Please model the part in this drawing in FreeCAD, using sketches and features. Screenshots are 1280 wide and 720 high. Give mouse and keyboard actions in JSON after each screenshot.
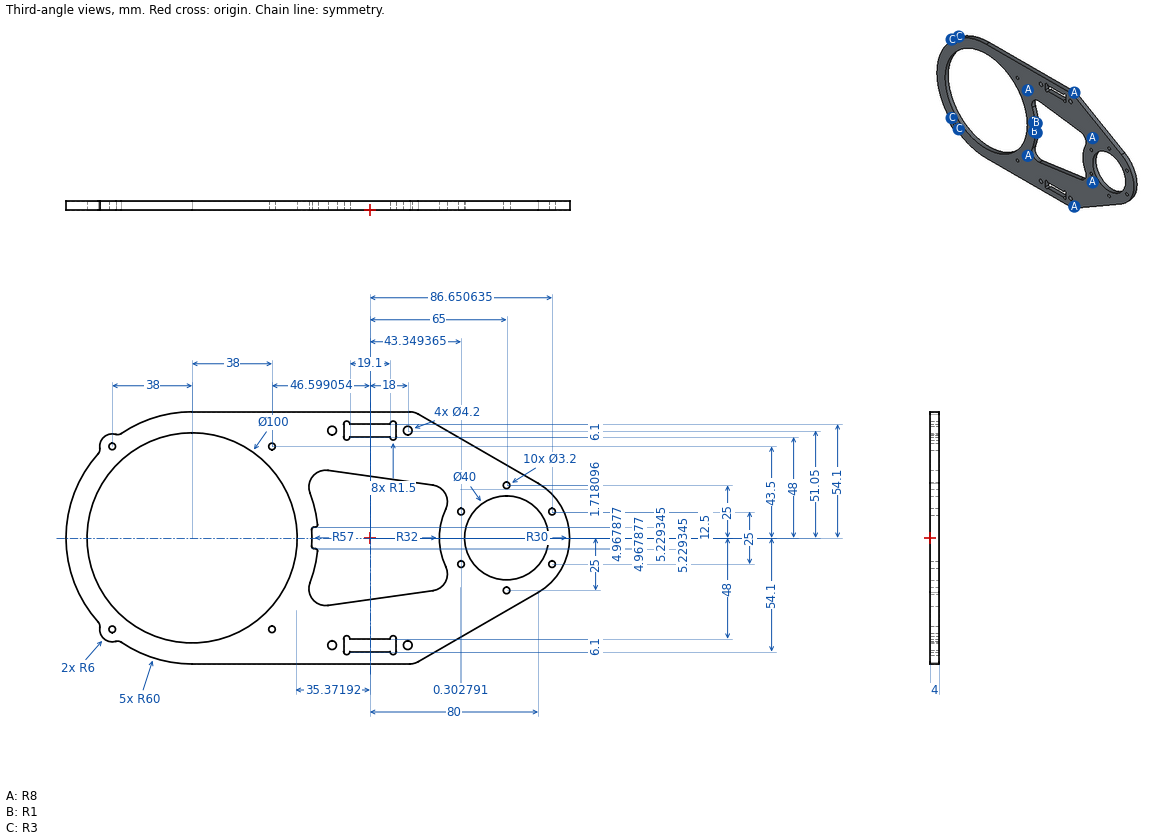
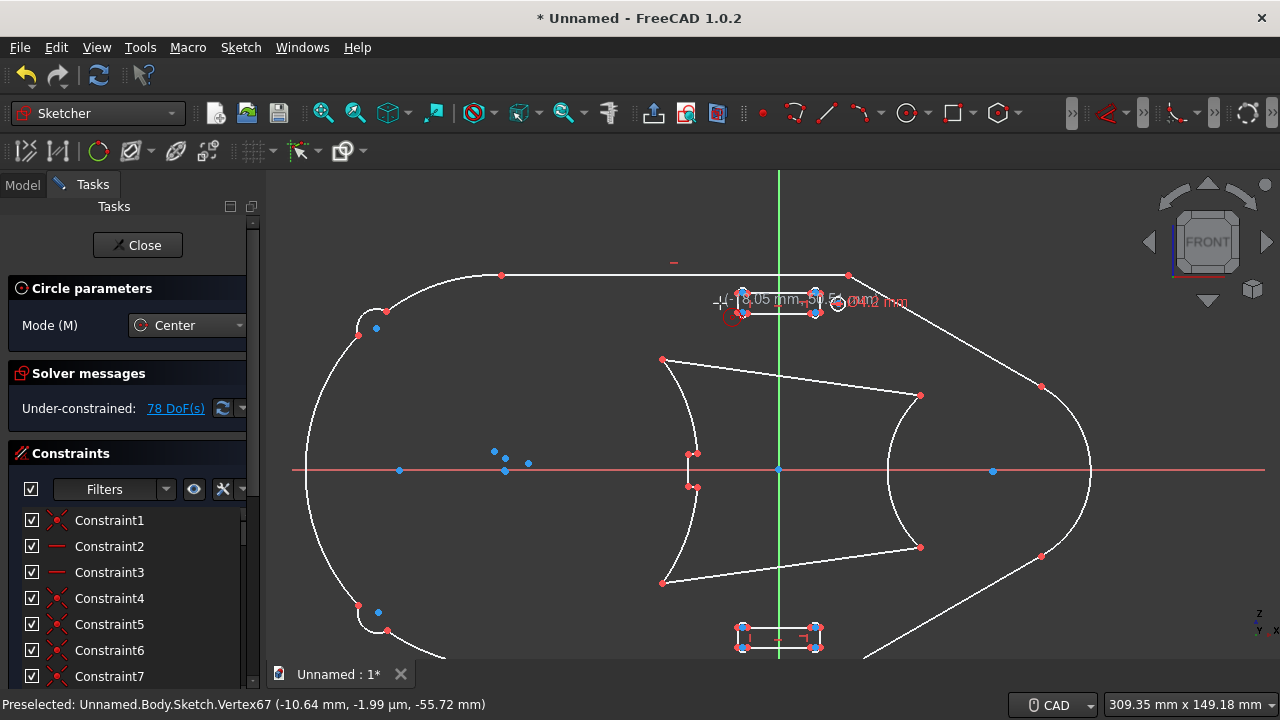
{"action": "left_click", "coordinate": [720, 303]}
{"action": "mouse_move", "coordinate": [715, 298]}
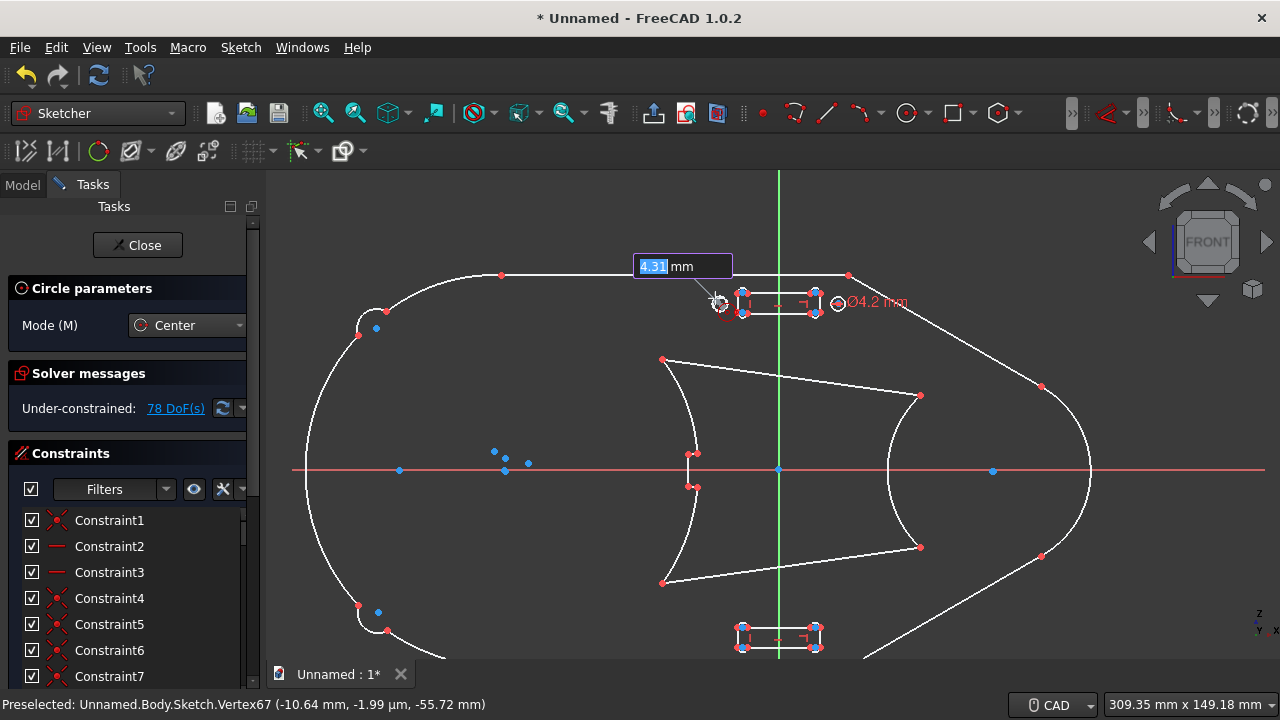
{"action": "type", "text": "4.2"}
{"action": "key", "text": "Return"}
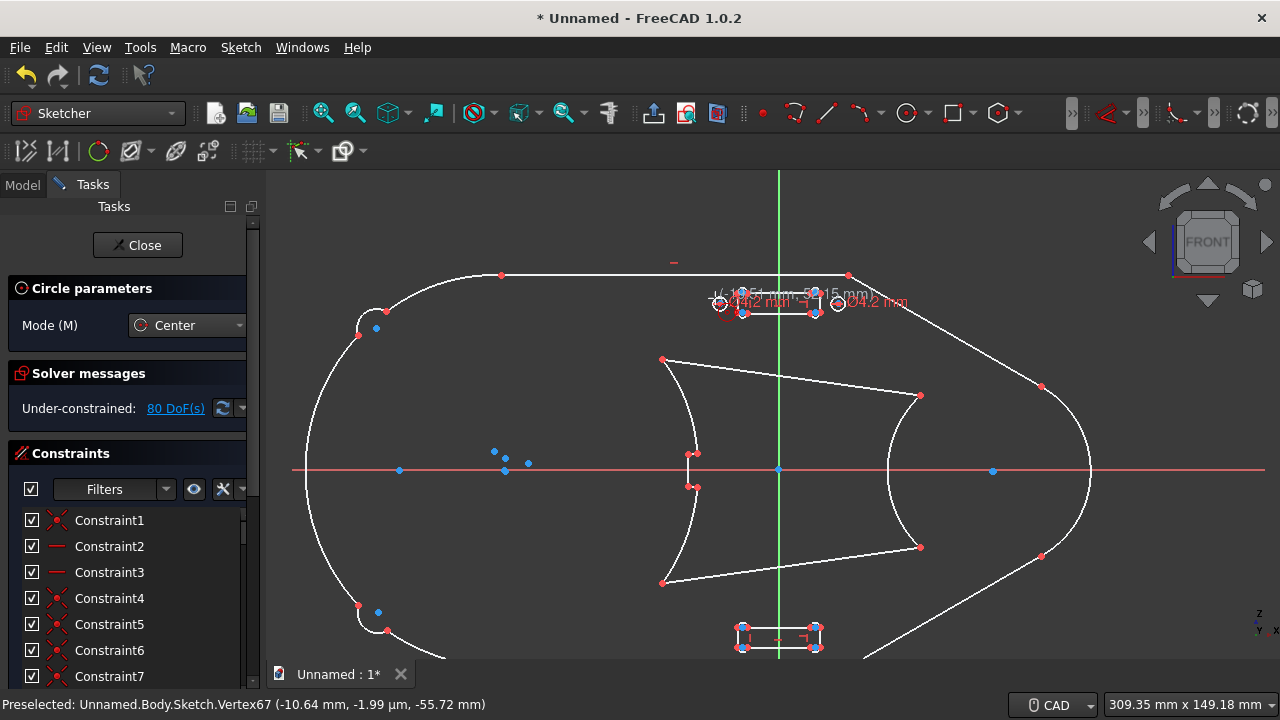
{"action": "scroll", "coordinate": [992, 388], "scroll_direction": "up", "scroll_amount": 8}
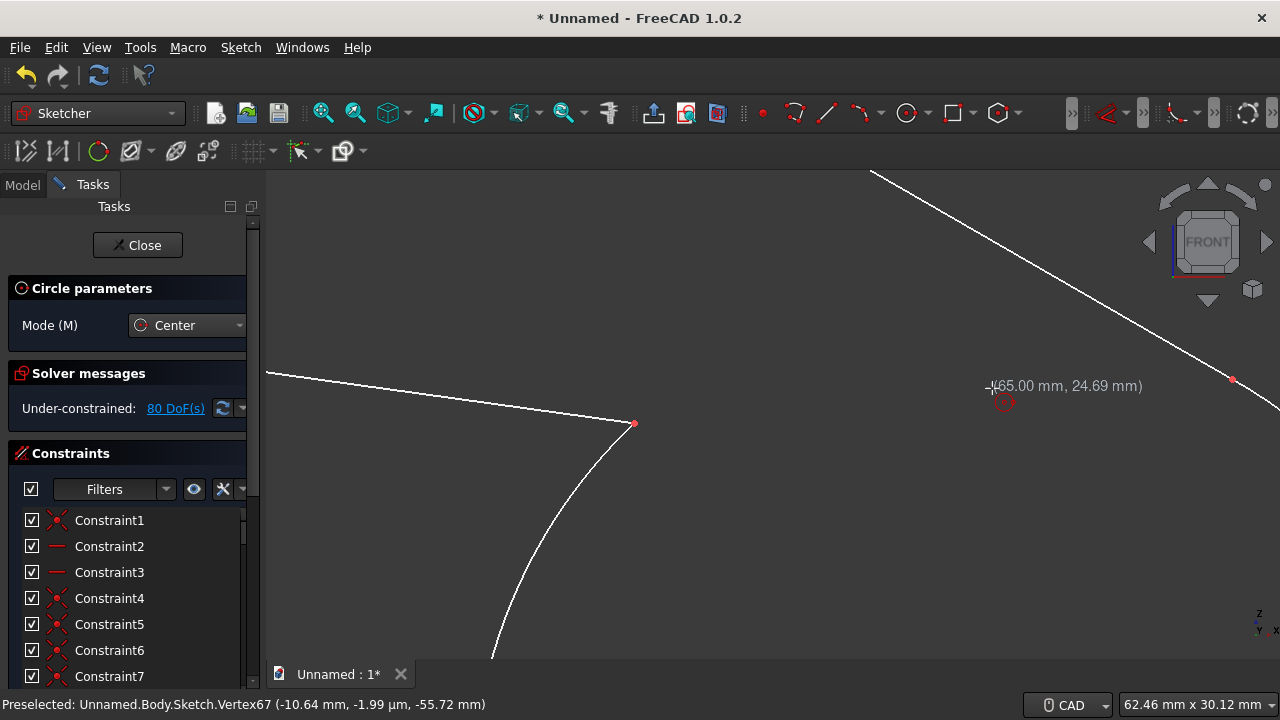
{"action": "scroll", "coordinate": [888, 355], "scroll_direction": "down", "scroll_amount": 10}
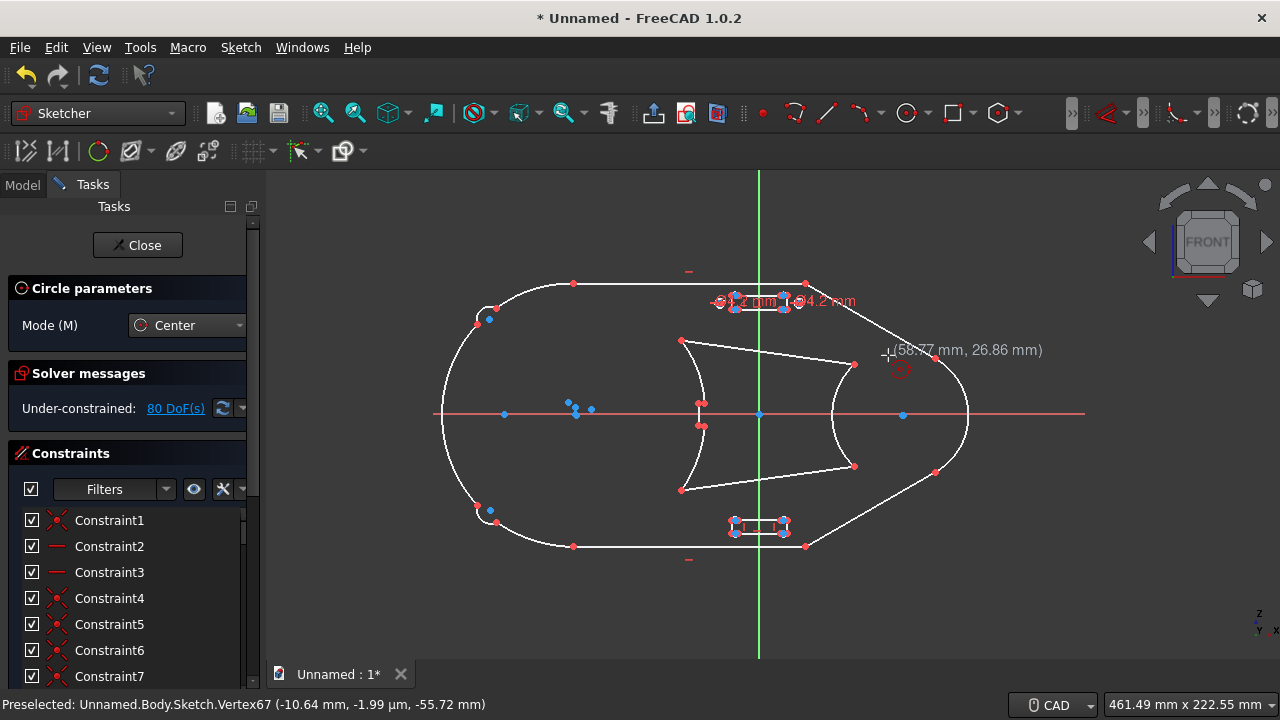
{"action": "left_click", "coordinate": [902, 360]}
{"action": "mouse_move", "coordinate": [905, 357]}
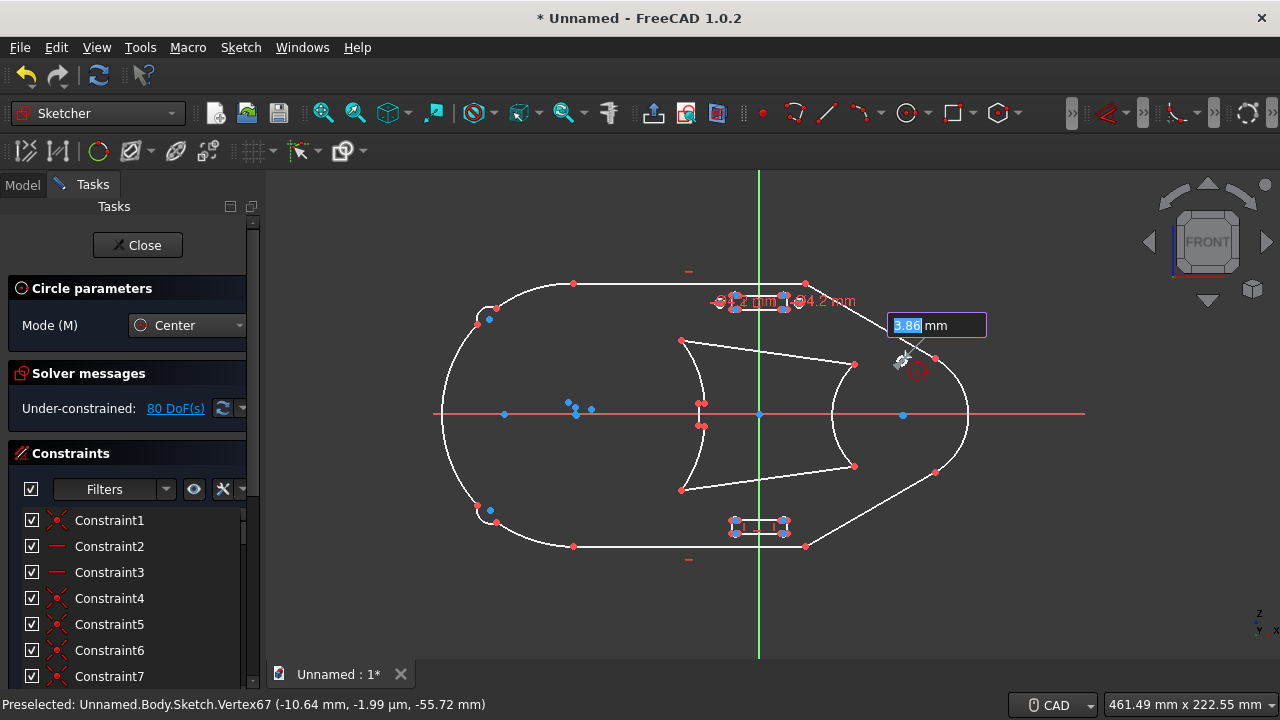
{"action": "type", "text": "3.2"}
{"action": "key", "text": "Return"}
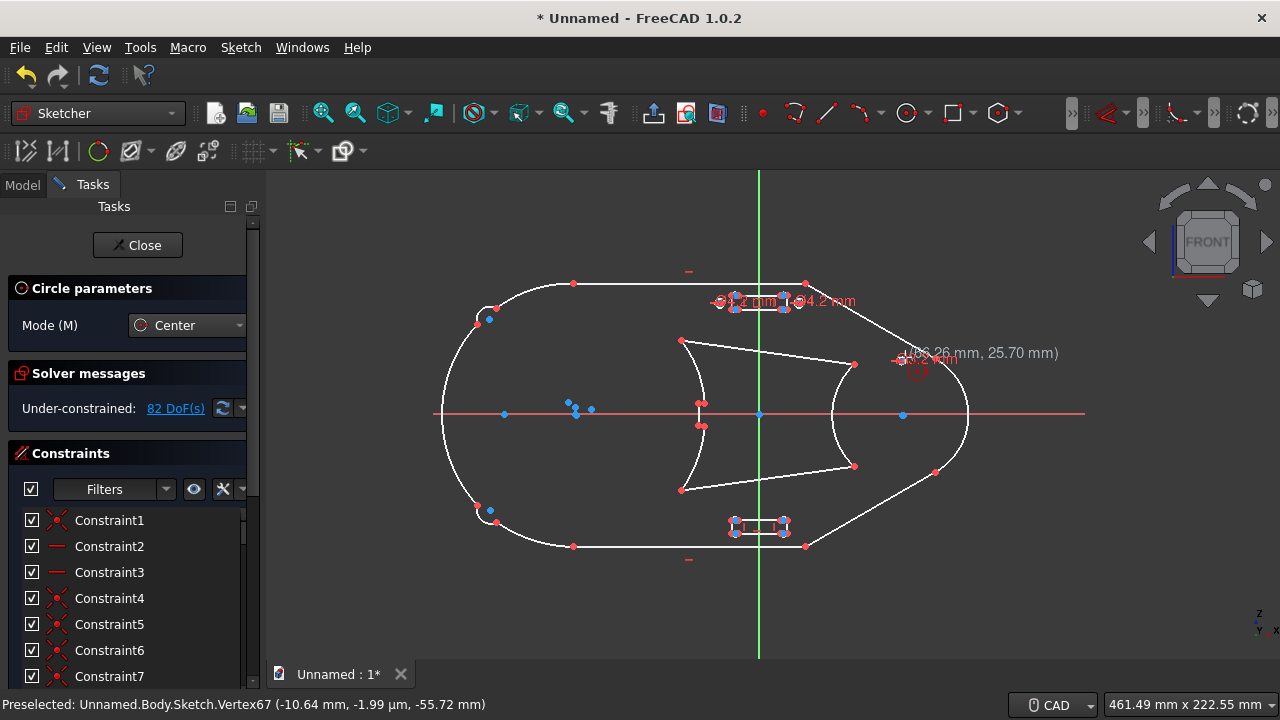
{"action": "scroll", "coordinate": [950, 387], "scroll_direction": "up", "scroll_amount": 10}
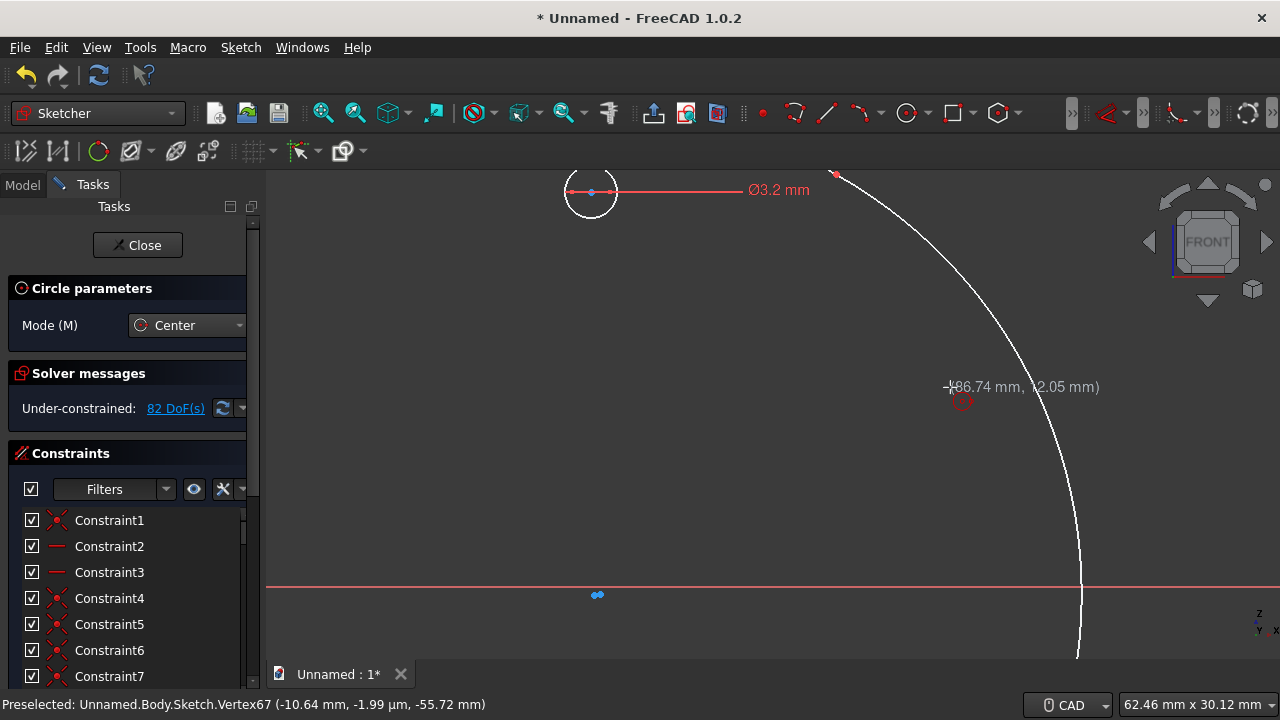
{"action": "scroll", "coordinate": [950, 387], "scroll_direction": "down", "scroll_amount": 10}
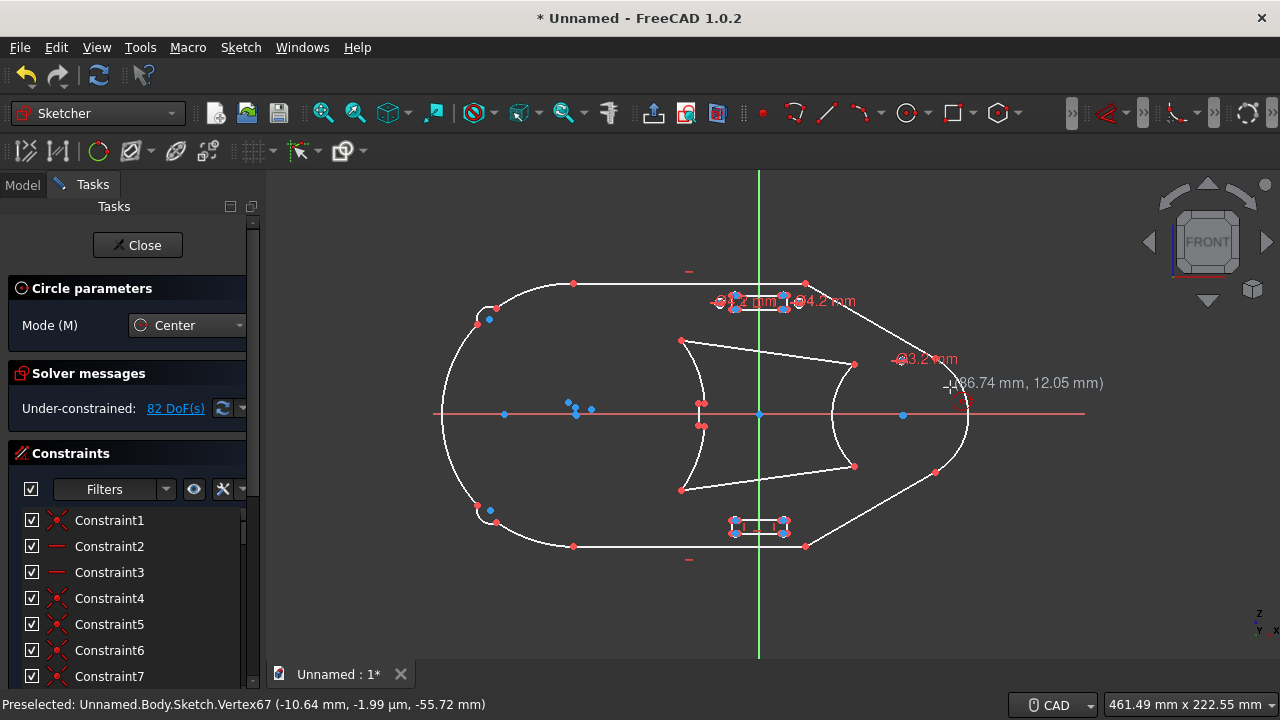
{"action": "scroll", "coordinate": [950, 387], "scroll_direction": "up", "scroll_amount": 2}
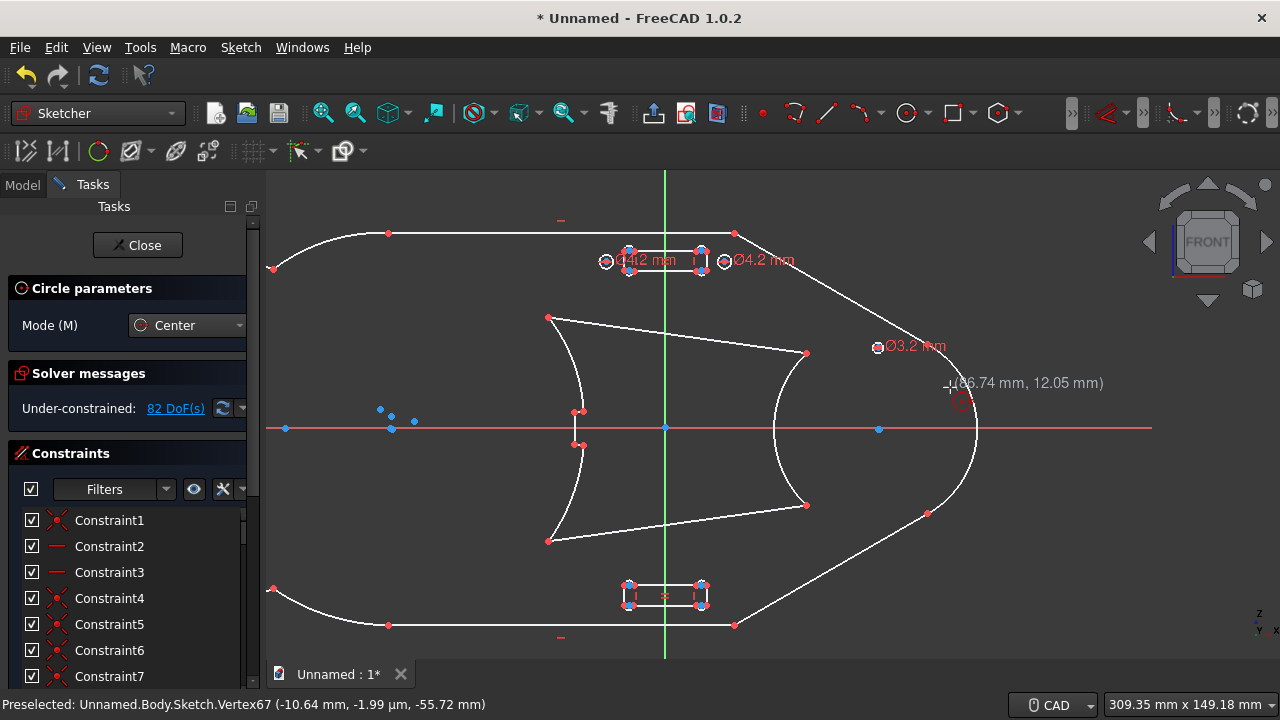
{"action": "left_click", "coordinate": [949, 387]}
{"action": "mouse_move", "coordinate": [946, 383]}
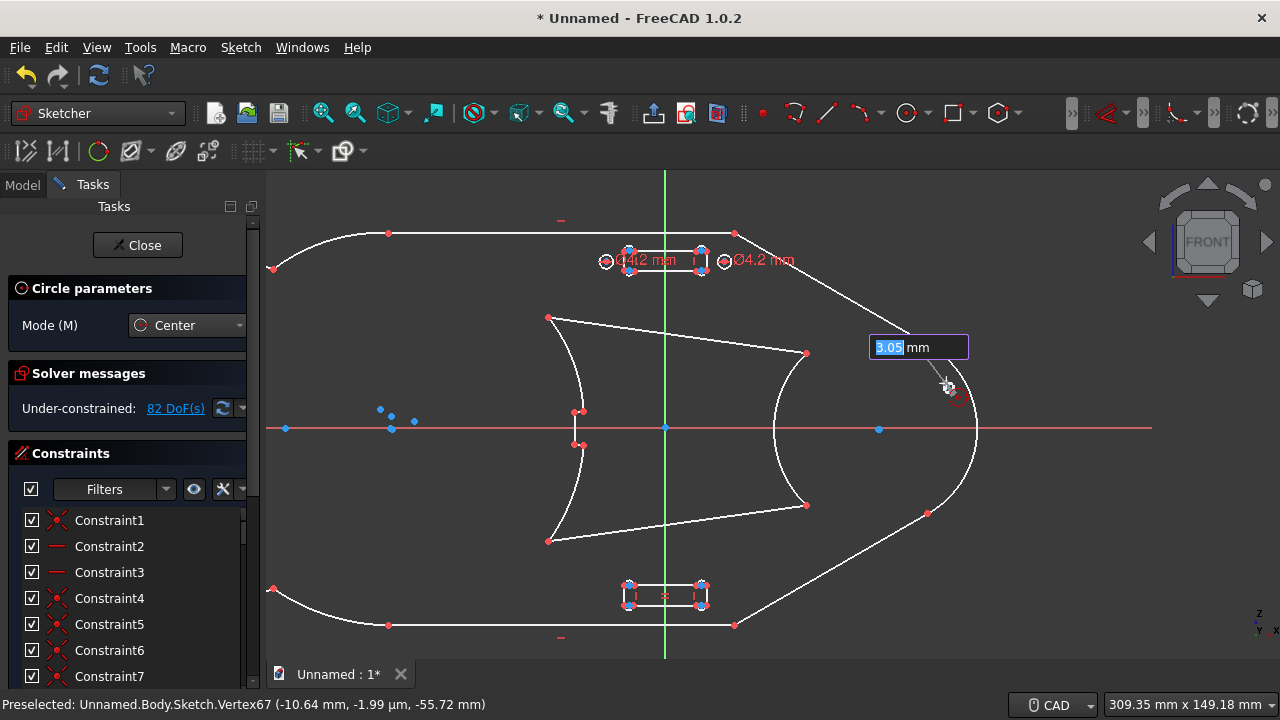
{"action": "type", "text": "3.2"}
{"action": "key", "text": "Return"}